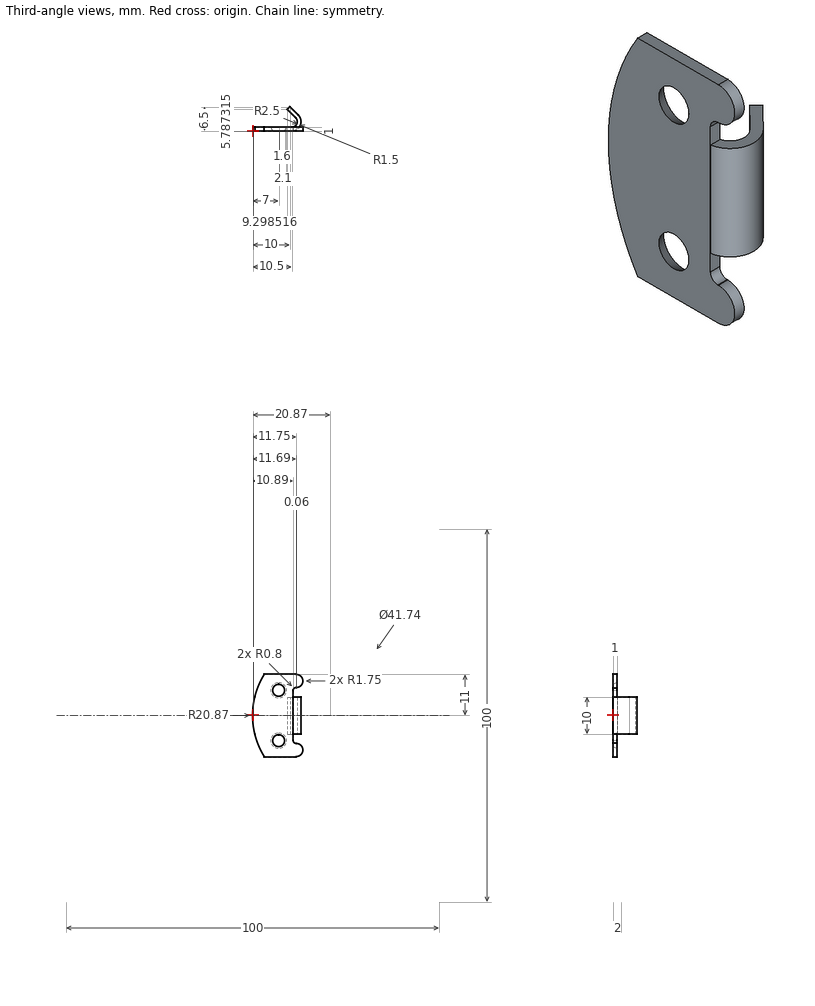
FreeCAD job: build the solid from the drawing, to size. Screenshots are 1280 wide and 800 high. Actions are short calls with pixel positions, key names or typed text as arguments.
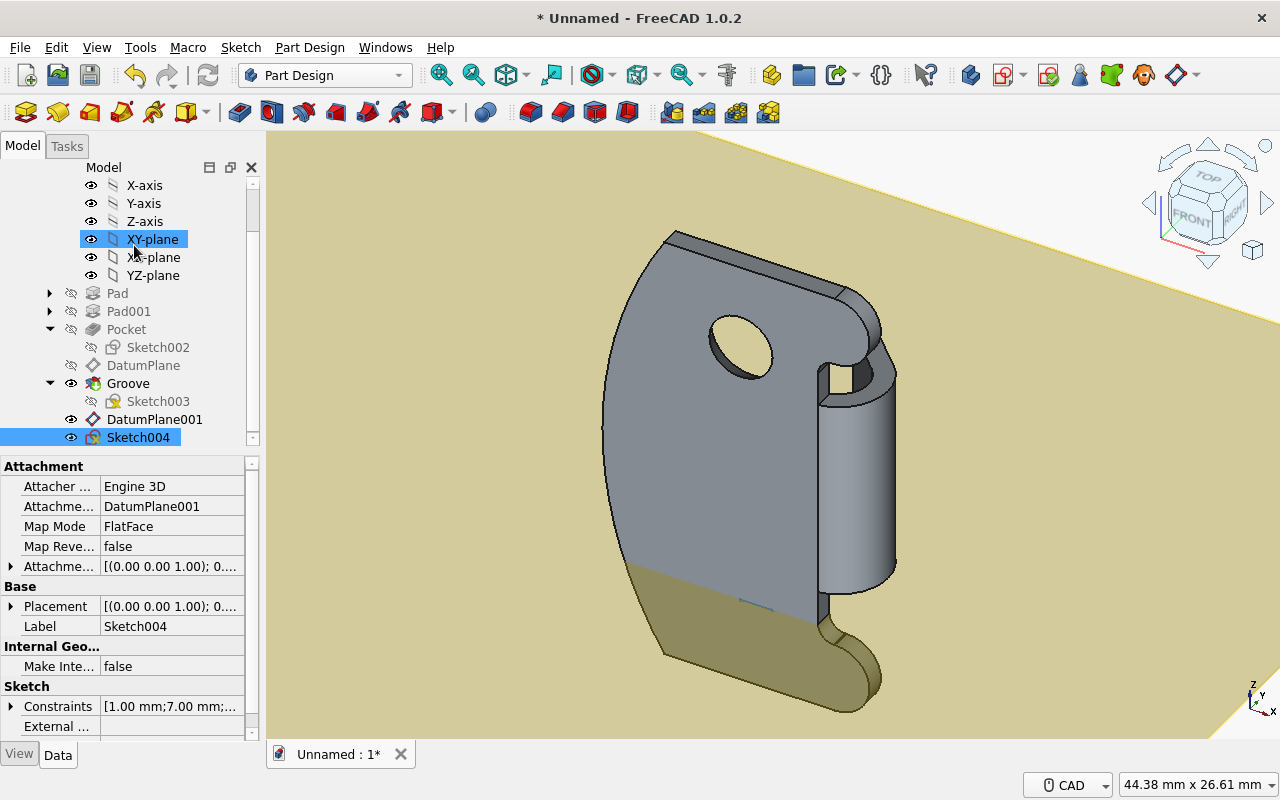
click(304, 112)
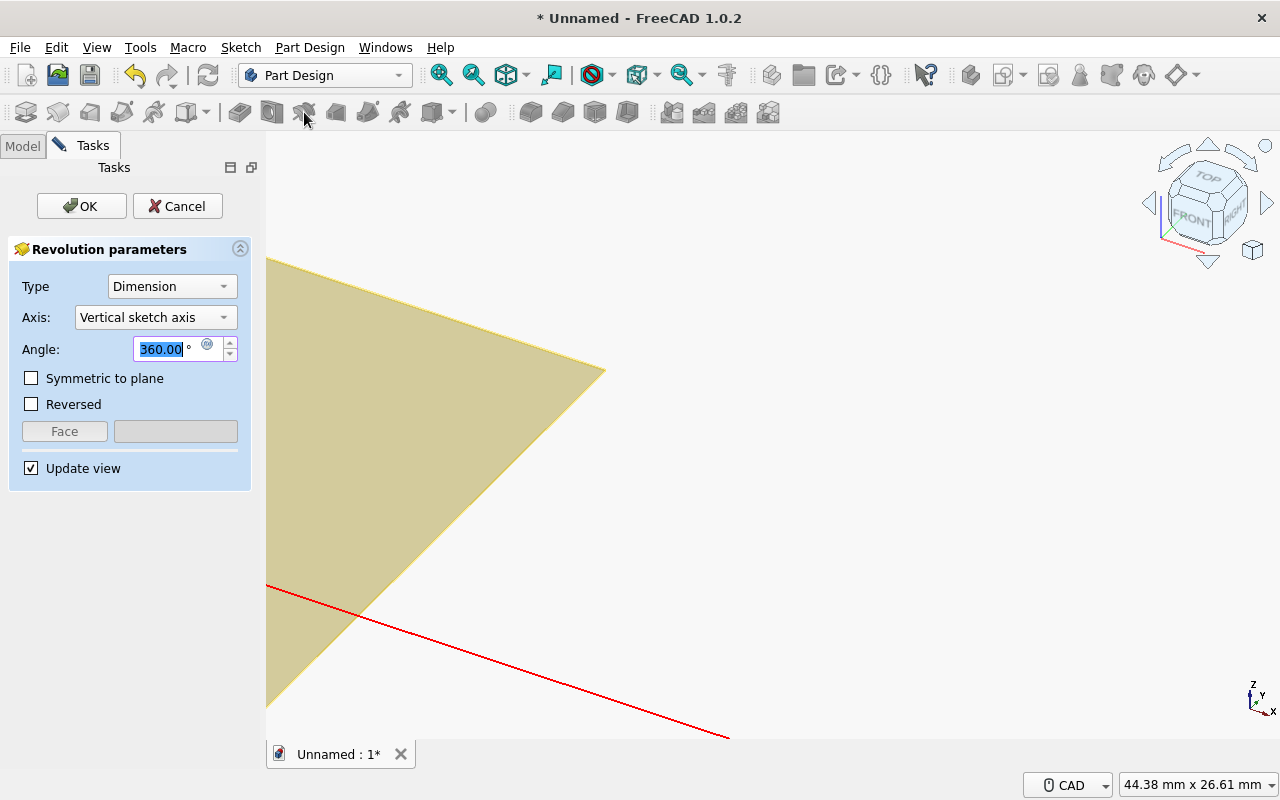
click(156, 318)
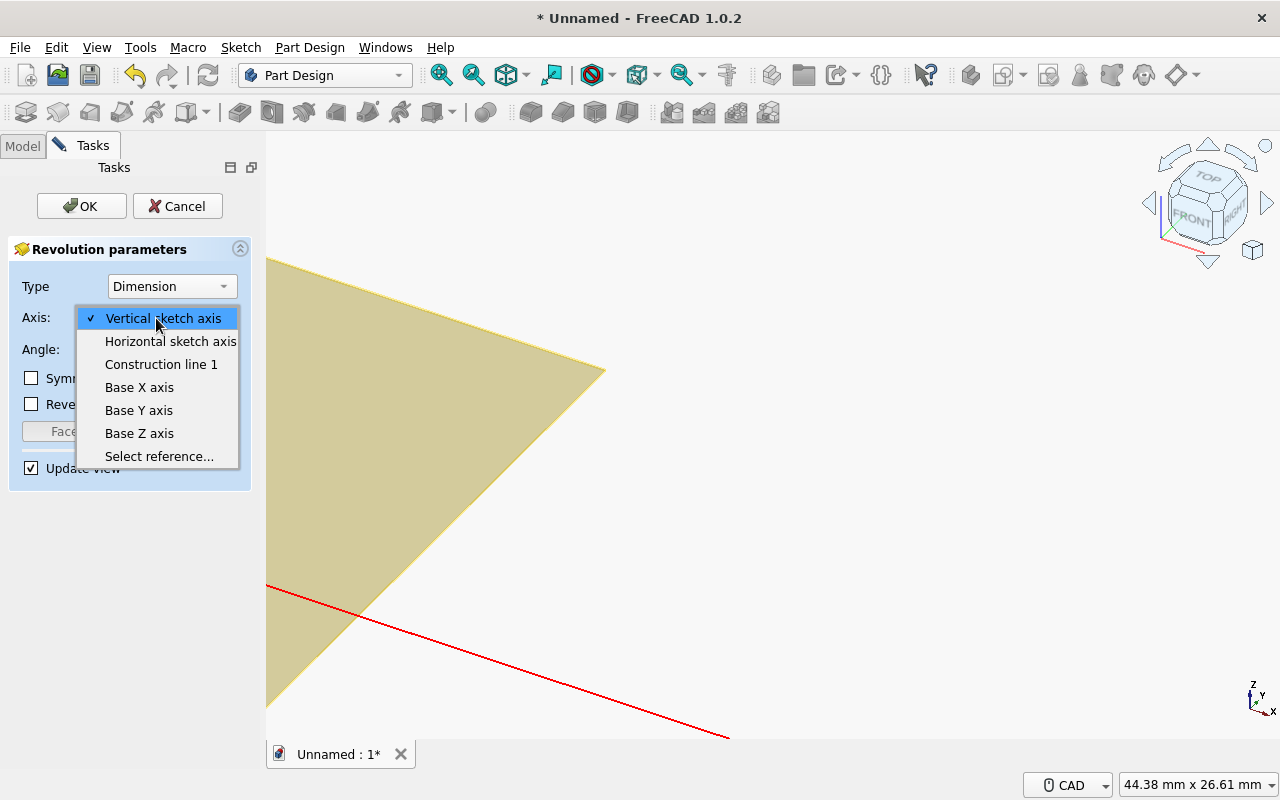
click(156, 364)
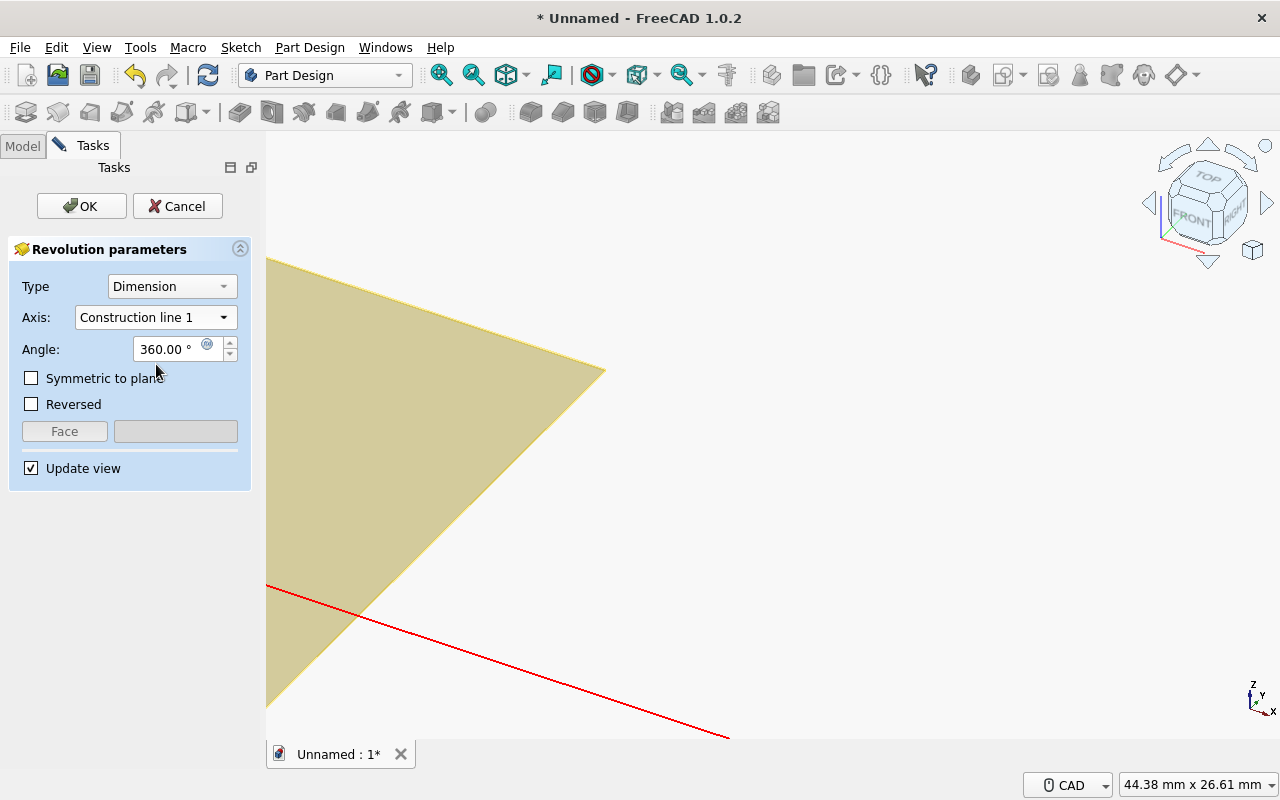
click(82, 206)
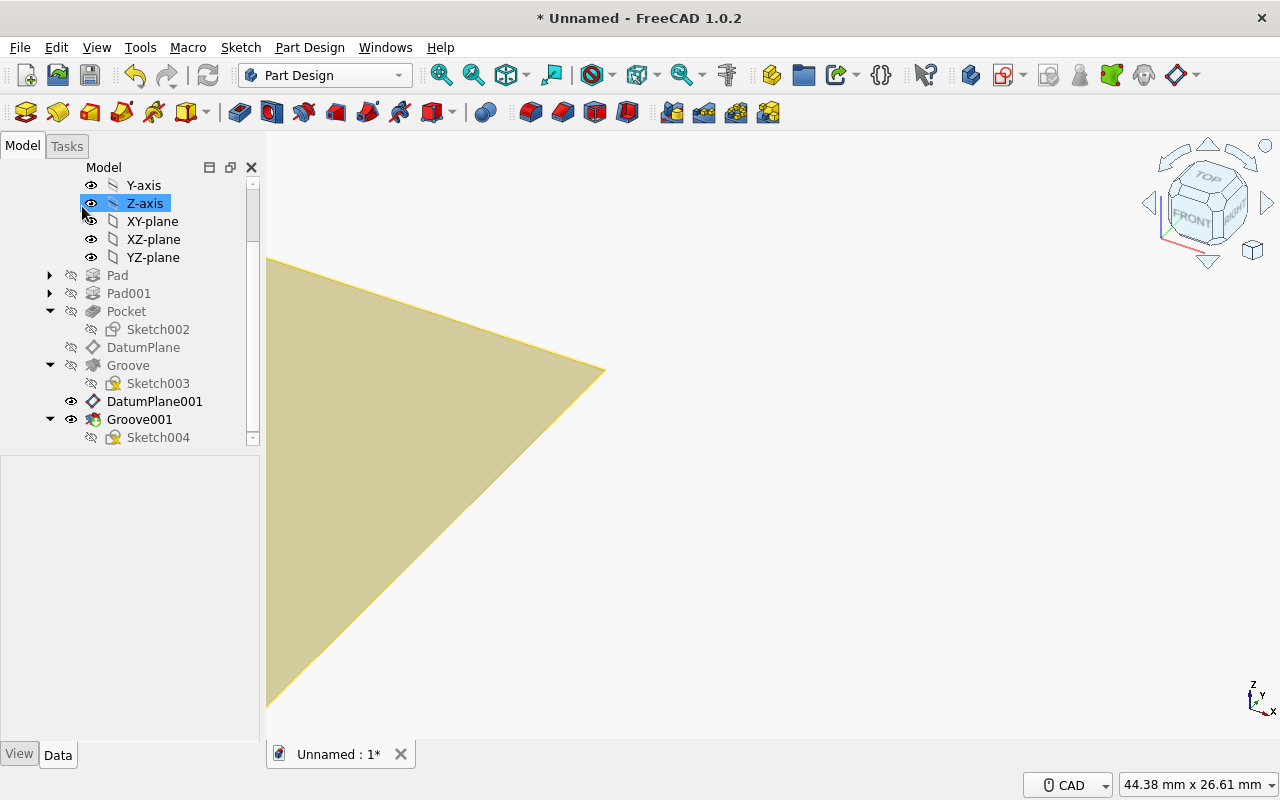
click(116, 401)
key(space)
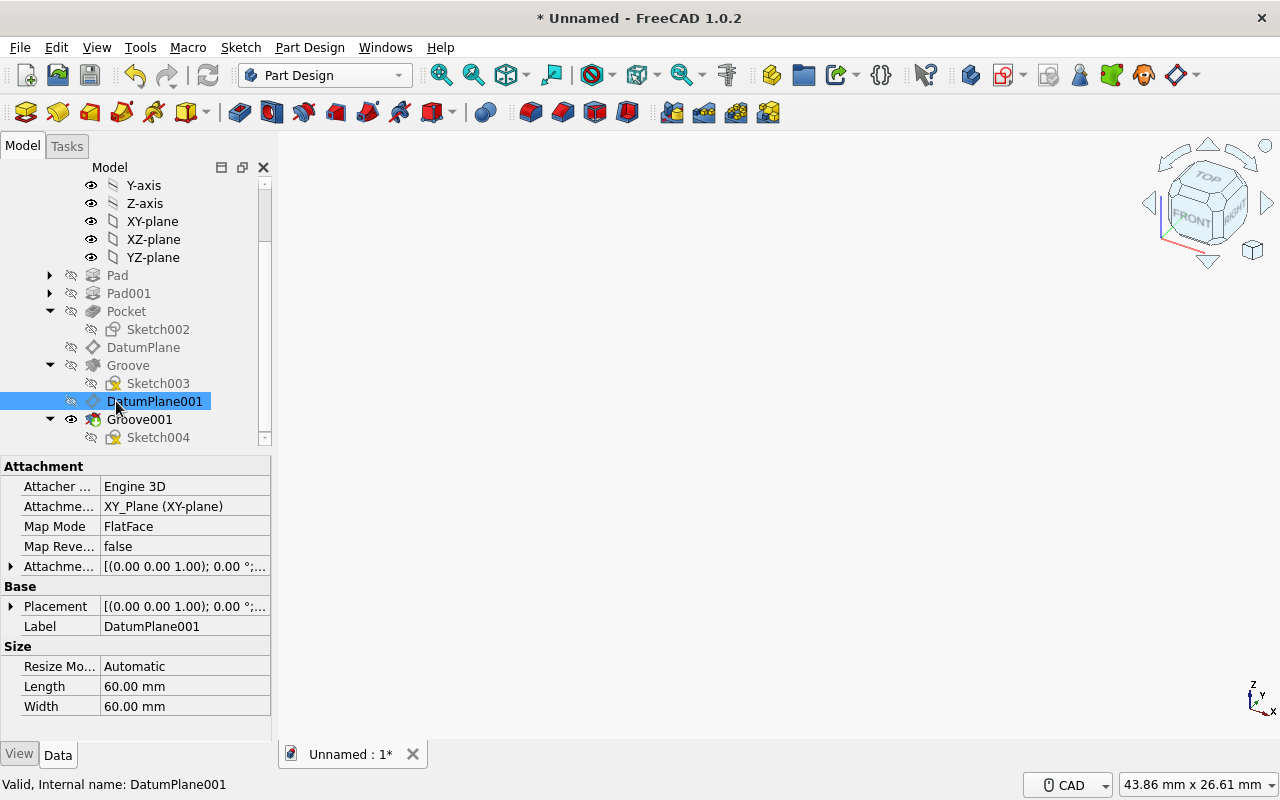
key(0)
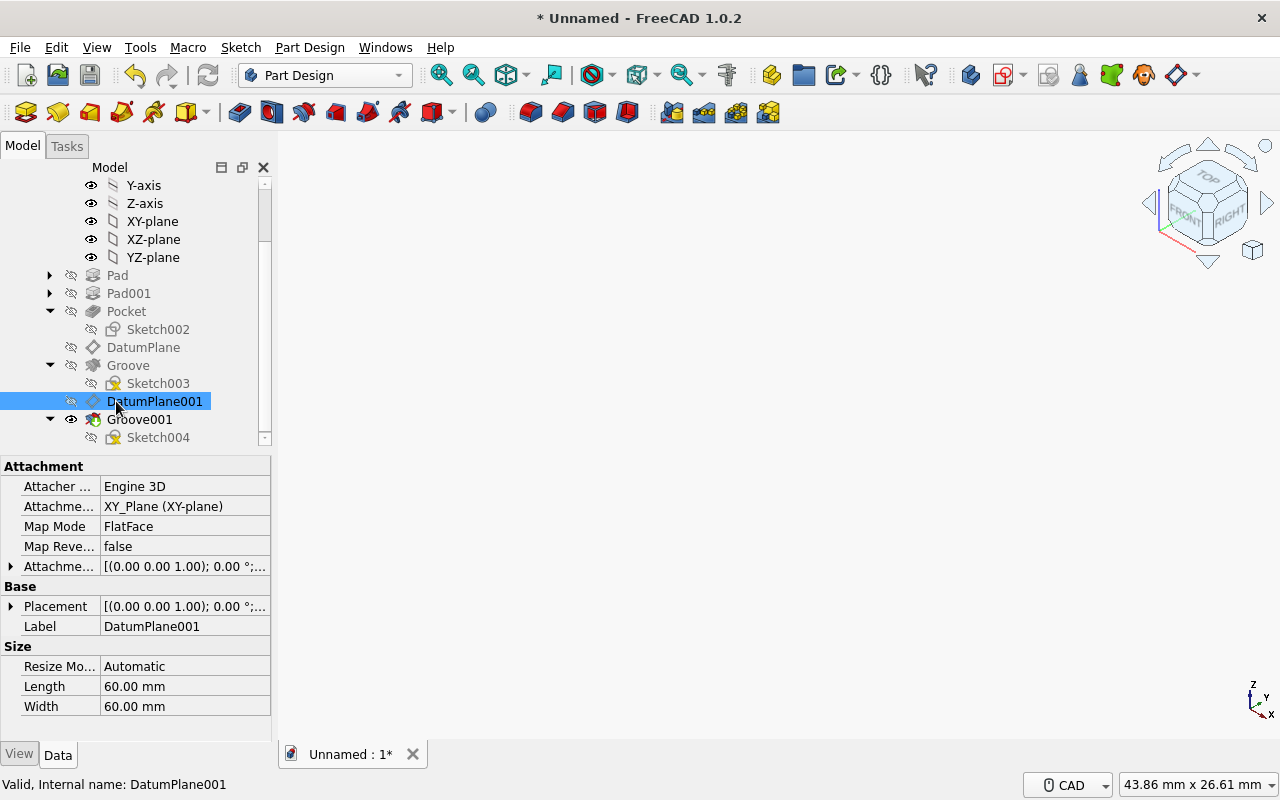
click(442, 76)